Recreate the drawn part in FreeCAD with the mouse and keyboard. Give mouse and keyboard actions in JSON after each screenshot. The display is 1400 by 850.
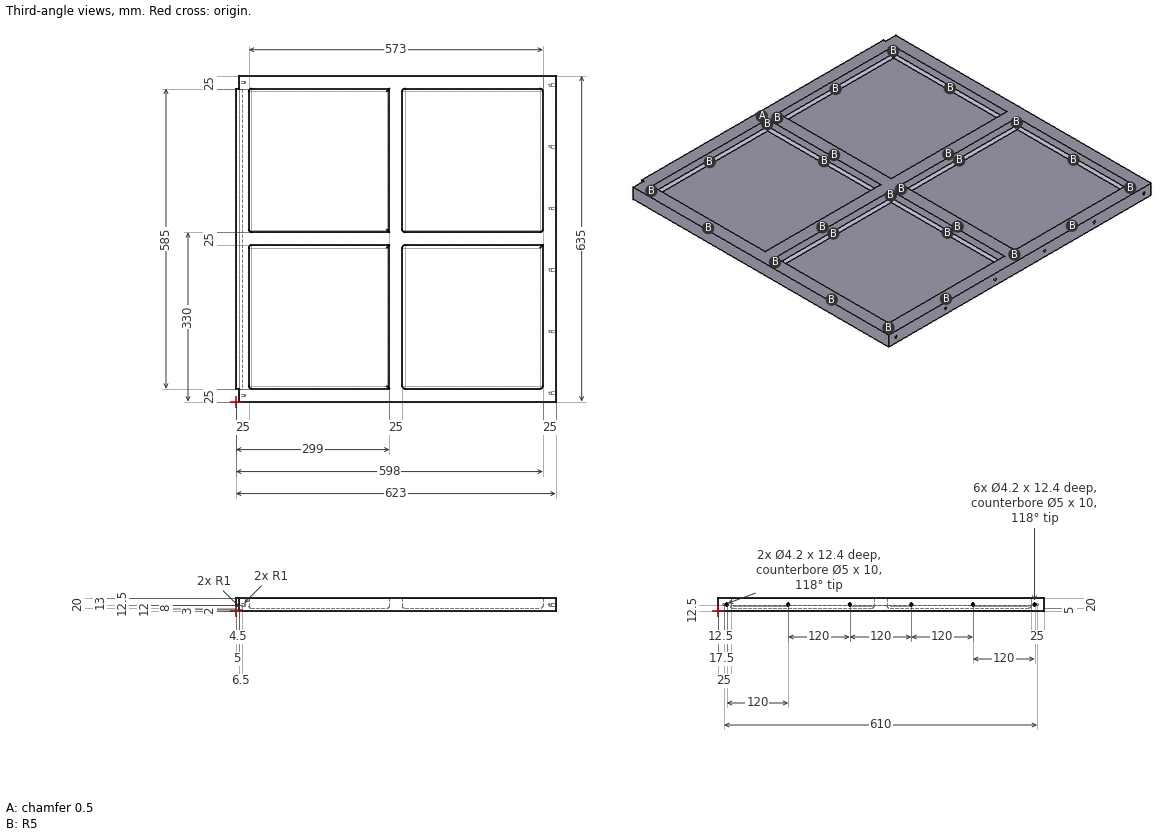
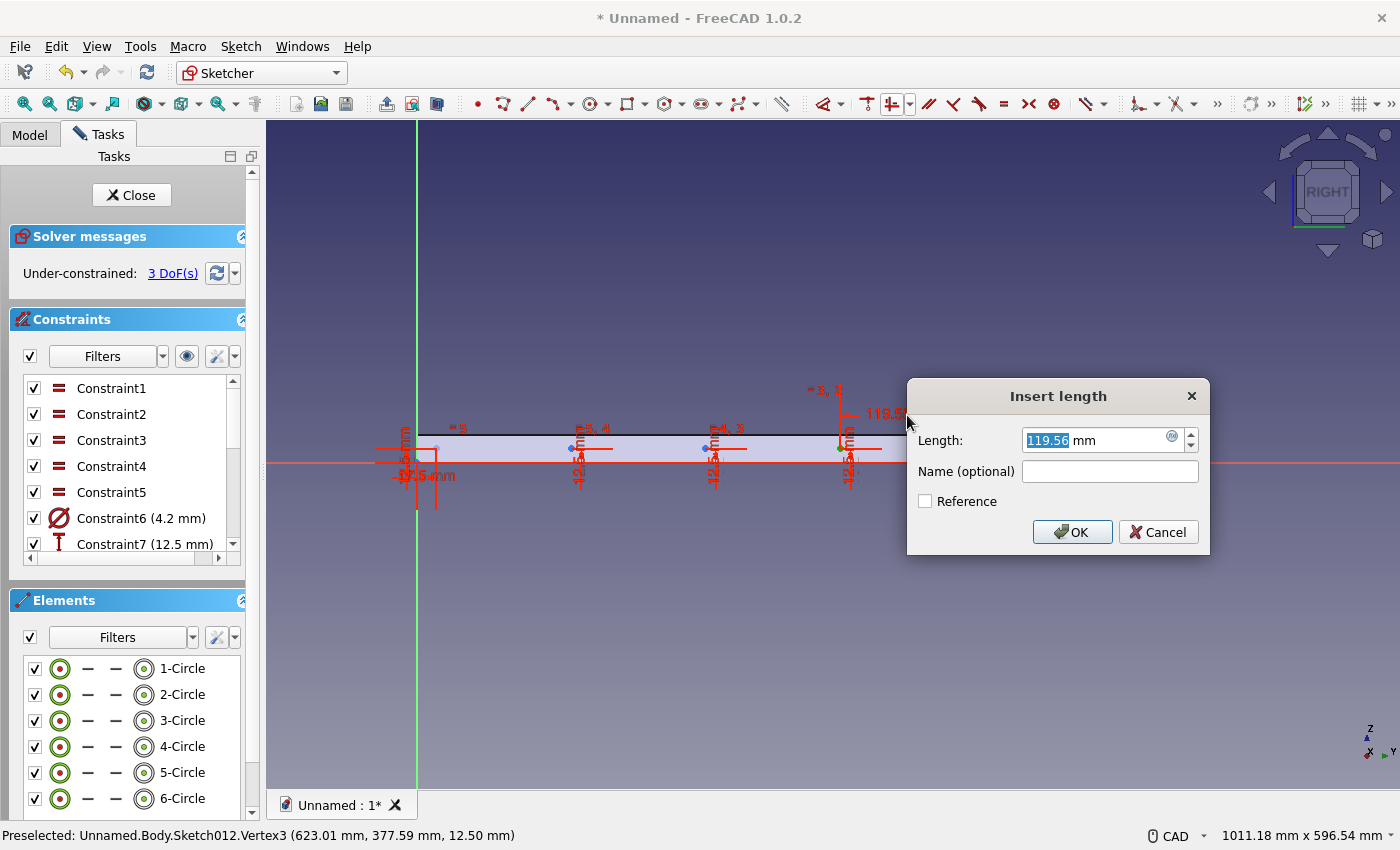
{"action": "type", "text": "120"}
{"action": "key", "text": "Return"}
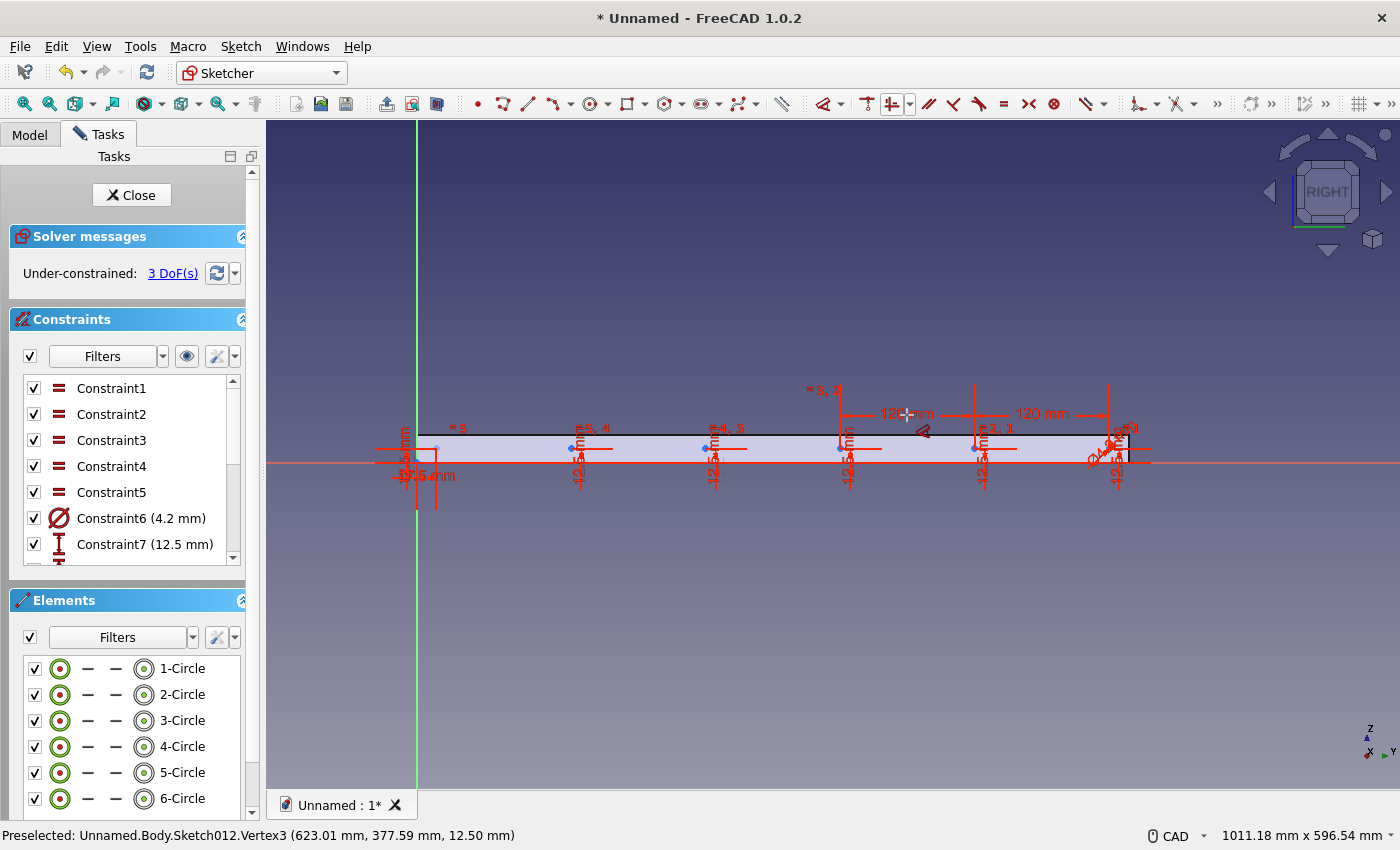
{"action": "left_click", "coordinate": [840, 449]}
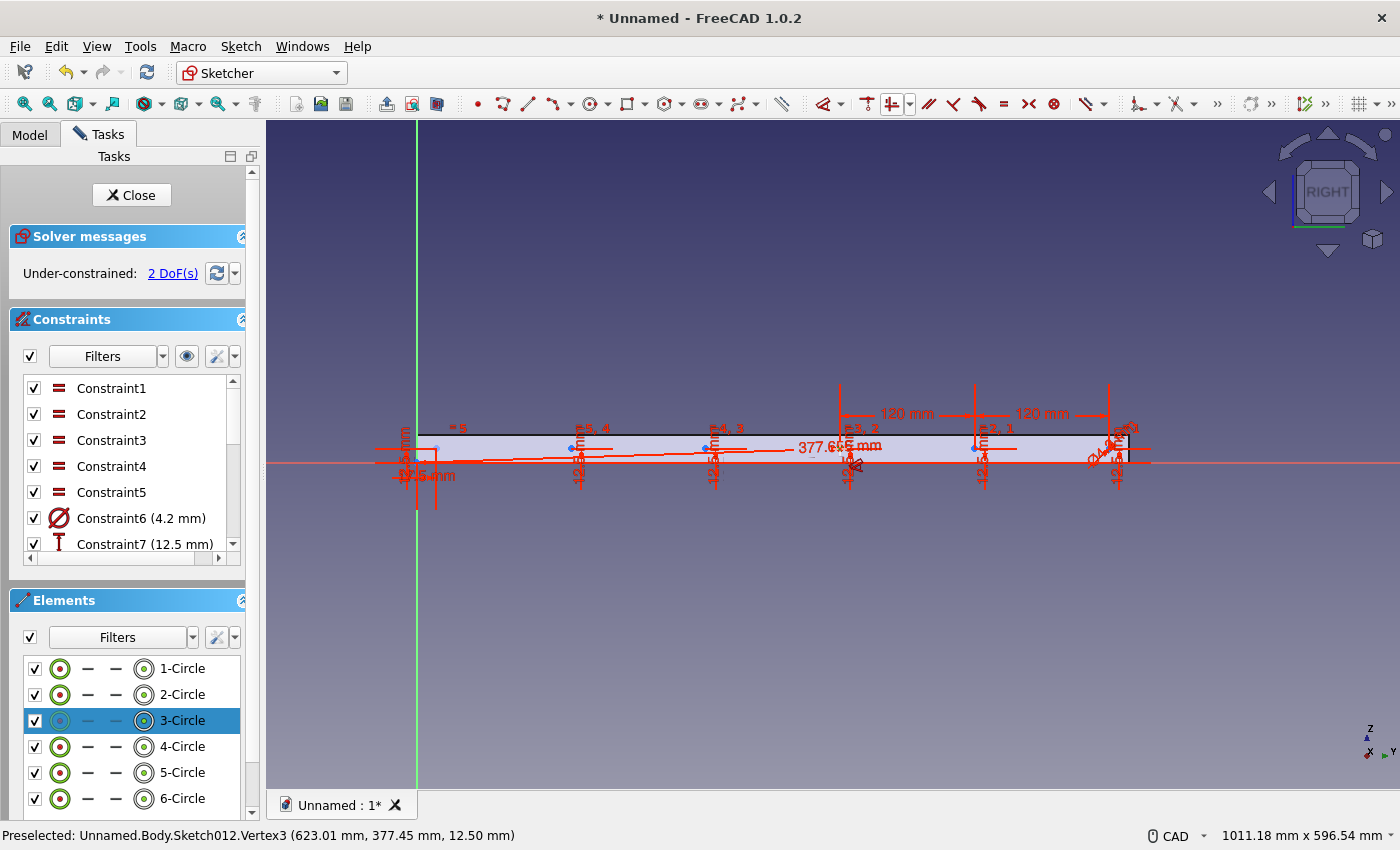
{"action": "left_click", "coordinate": [705, 449]}
{"action": "left_click", "coordinate": [773, 415]}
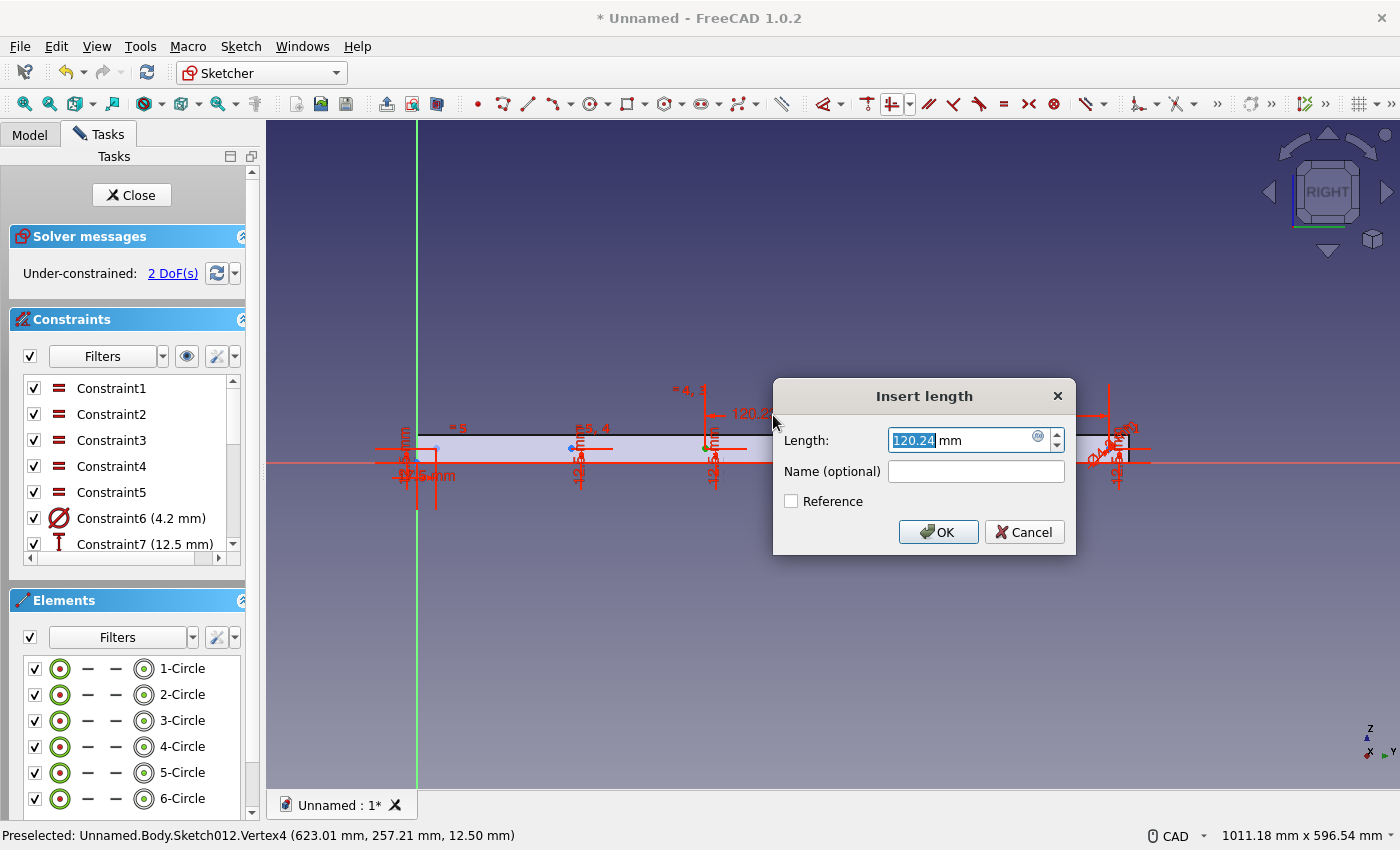
{"action": "type", "text": "120"}
{"action": "key", "text": "Return"}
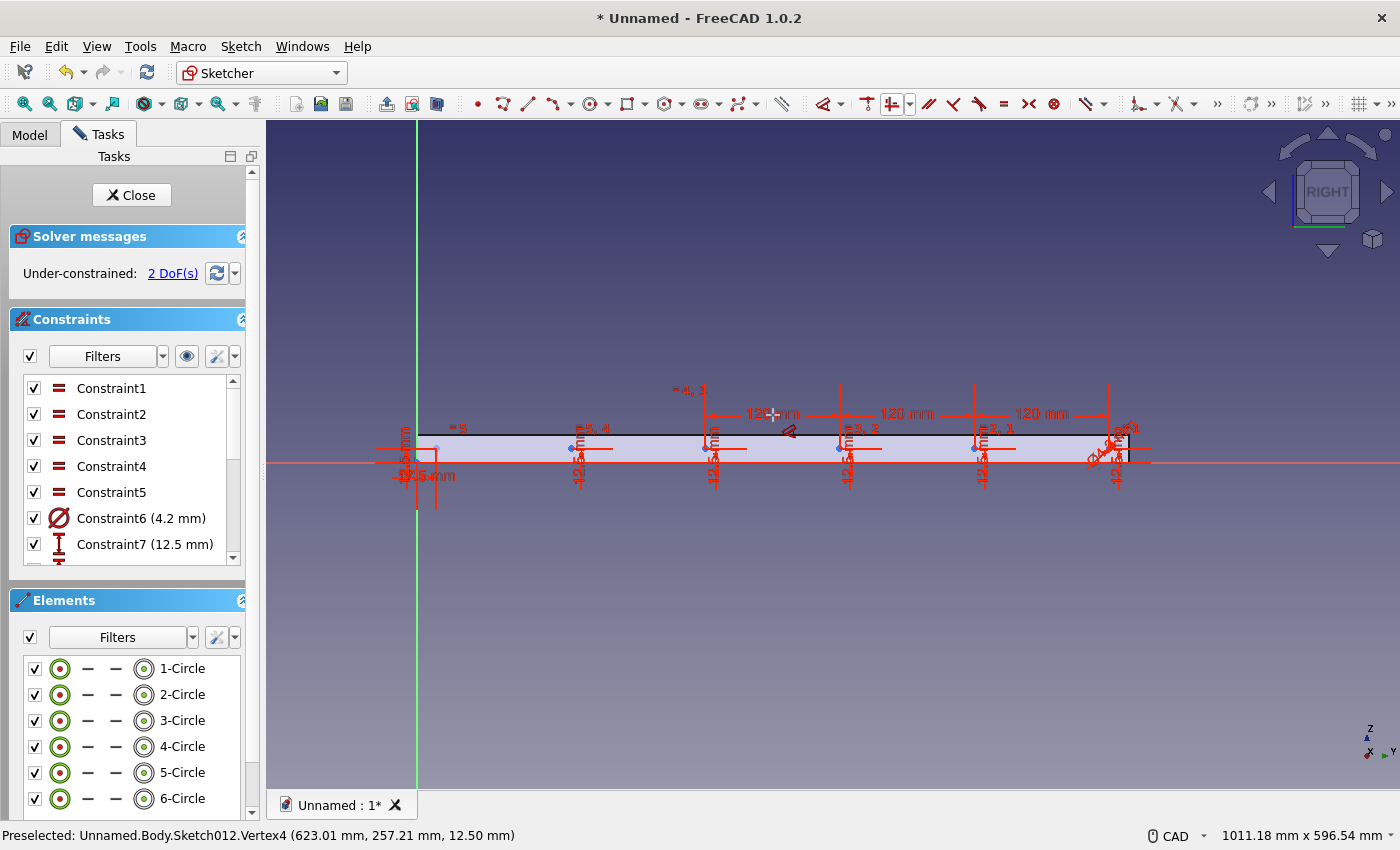
{"action": "left_click", "coordinate": [705, 449]}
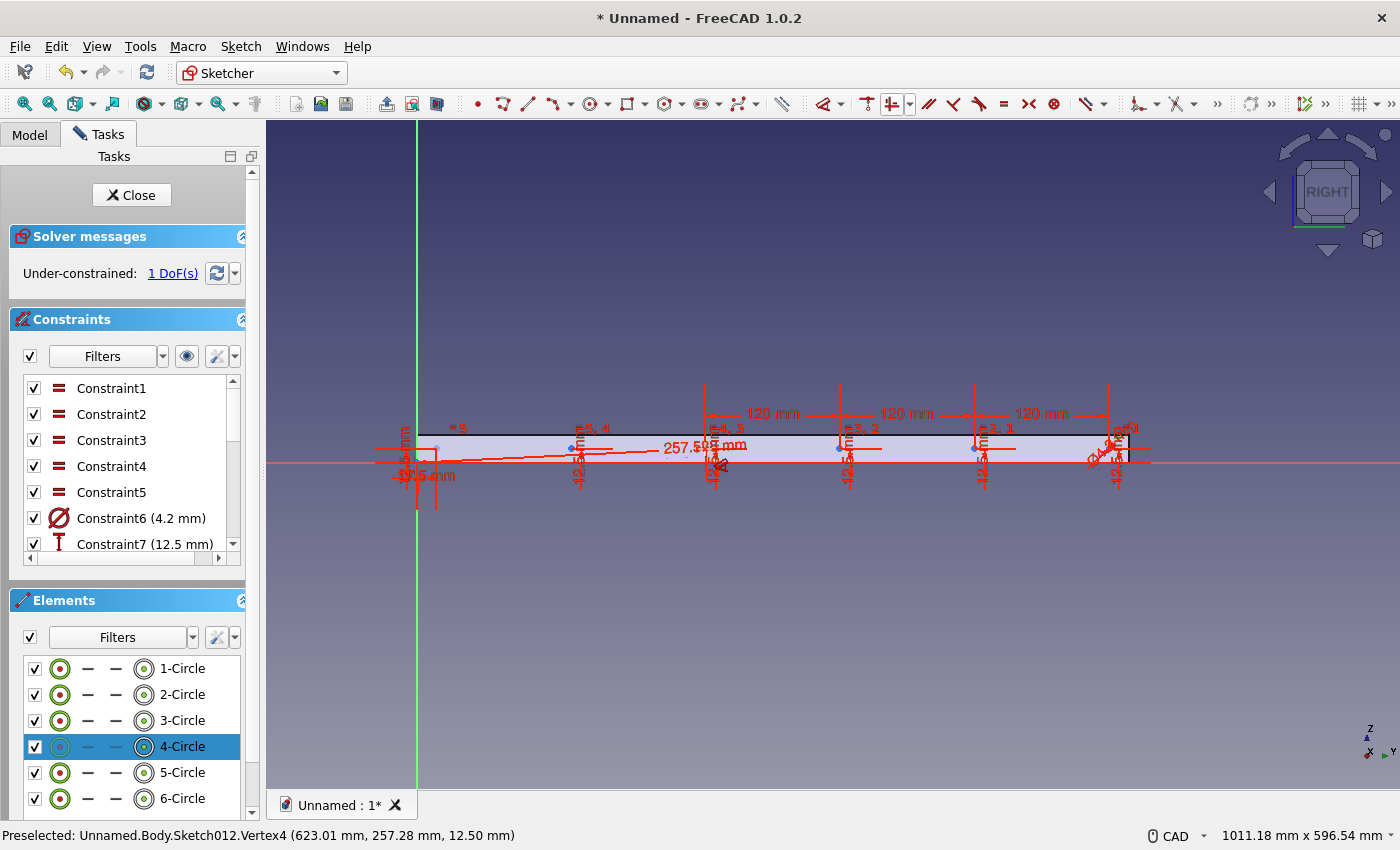
{"action": "left_click", "coordinate": [571, 449]}
{"action": "left_click", "coordinate": [638, 415]}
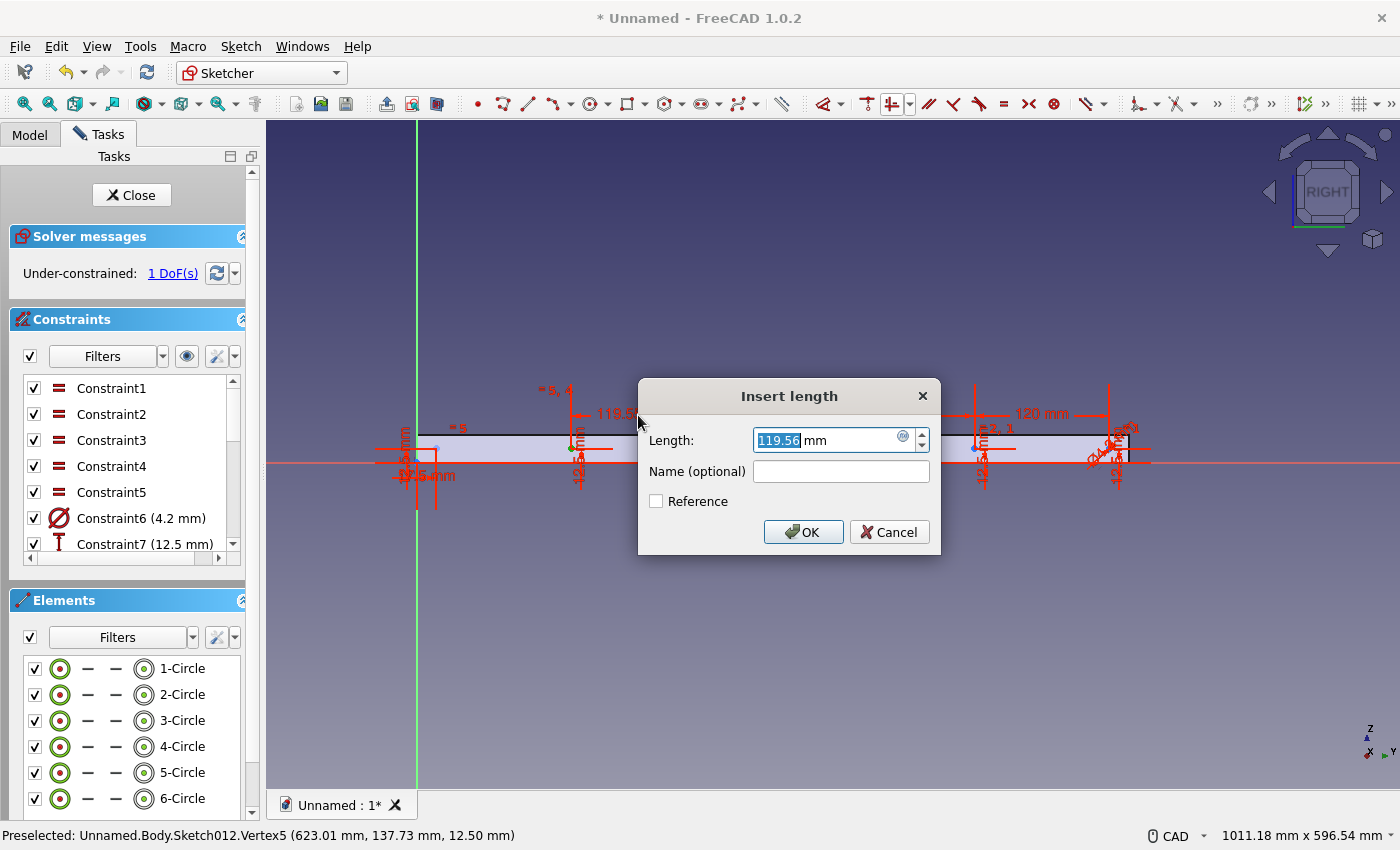
{"action": "type", "text": "120"}
{"action": "key", "text": "Return"}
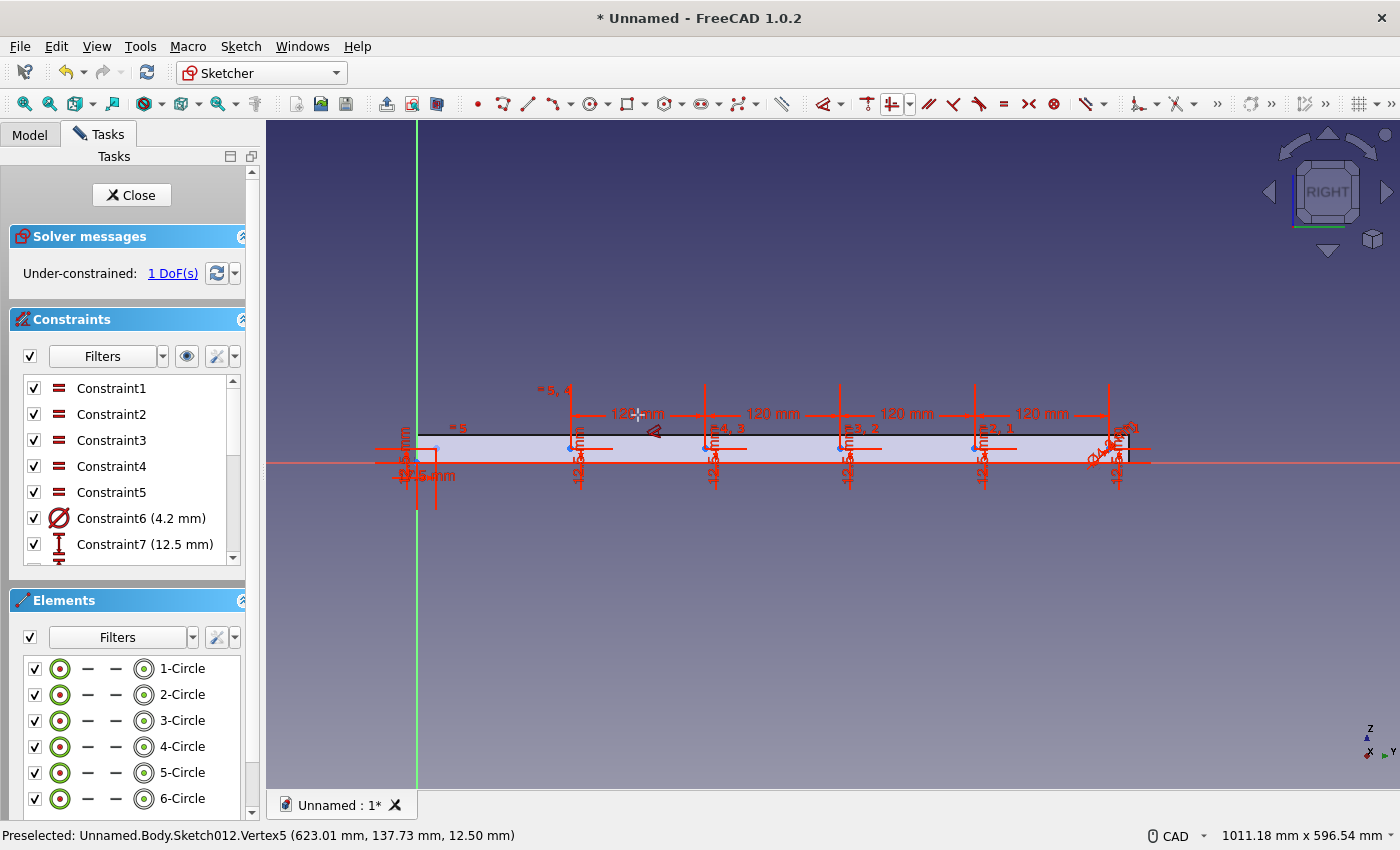
{"action": "left_click", "coordinate": [571, 449]}